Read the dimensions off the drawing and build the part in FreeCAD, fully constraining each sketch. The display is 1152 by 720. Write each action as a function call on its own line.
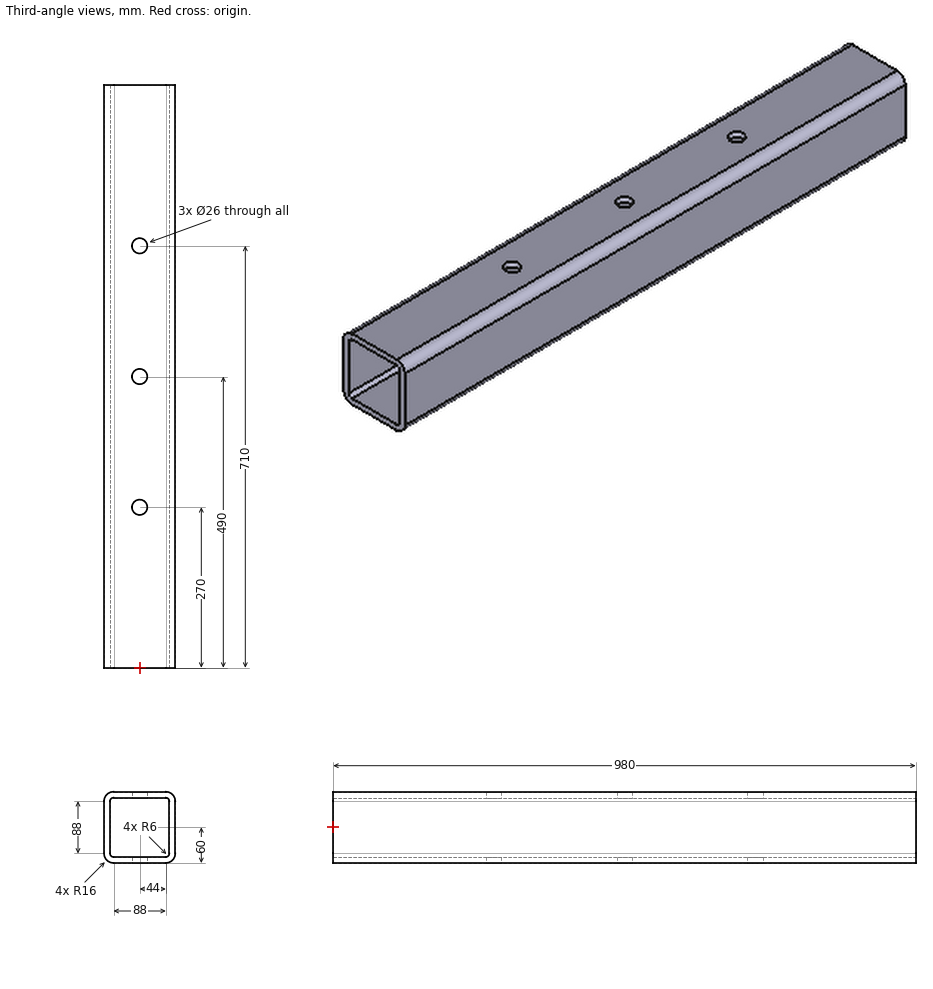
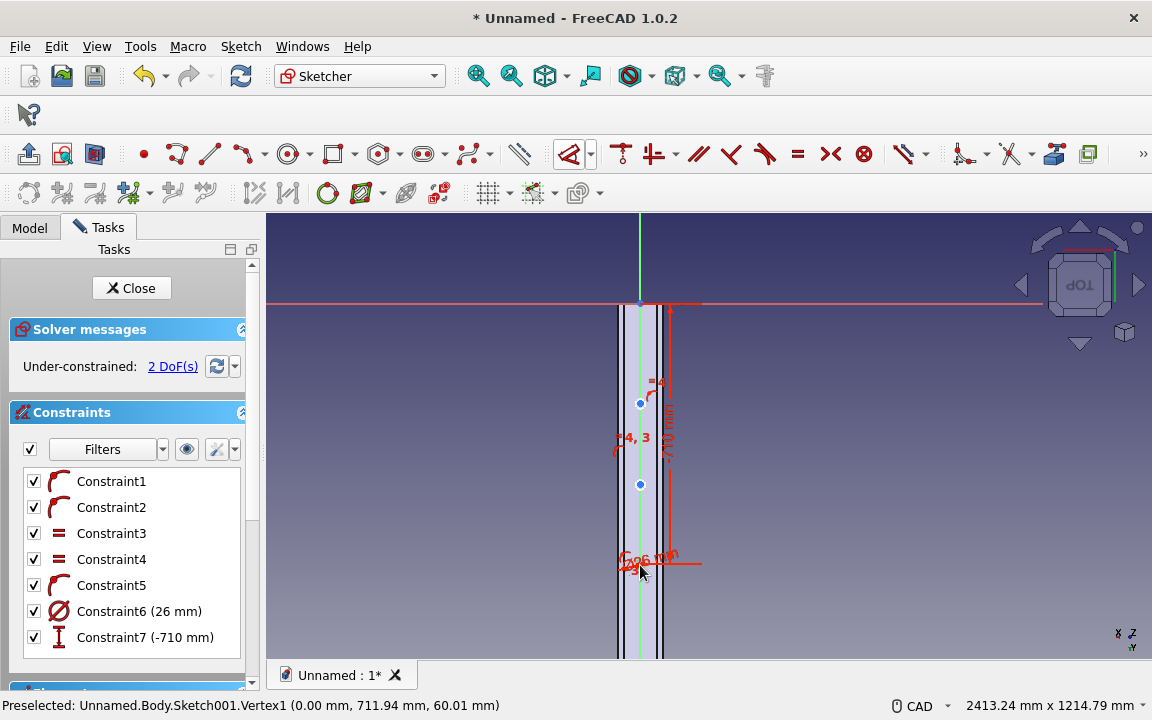
click(640, 485)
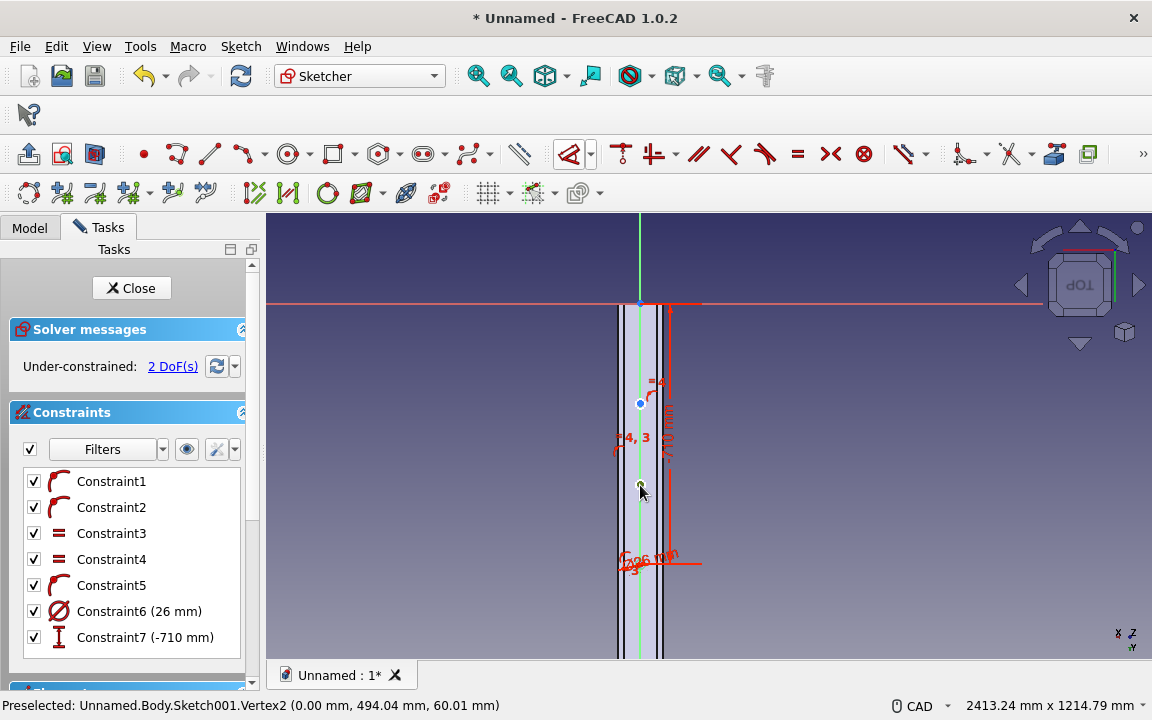
key(i)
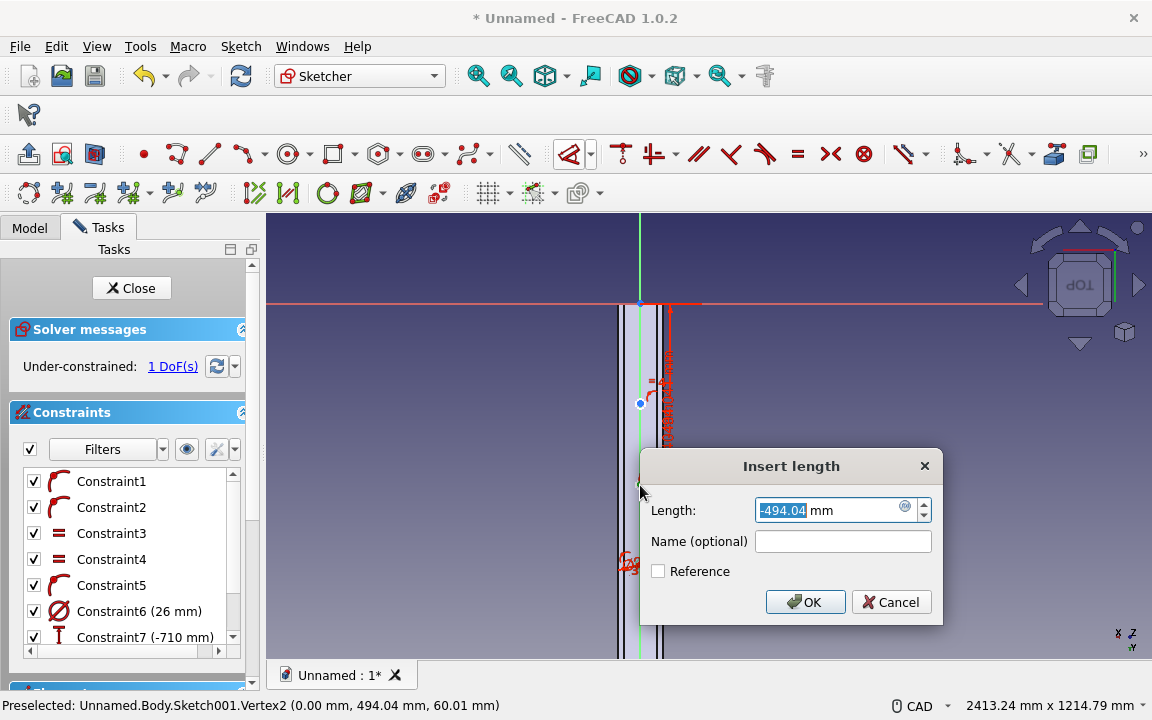
text(-490)
key(Return)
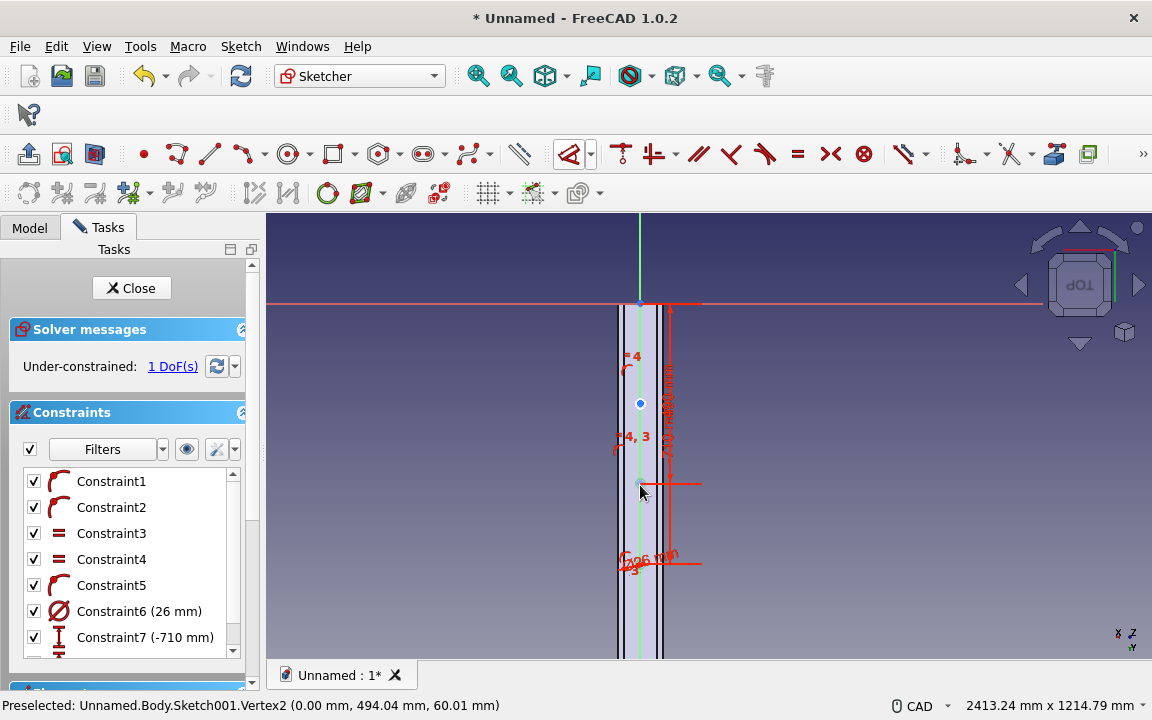
click(640, 404)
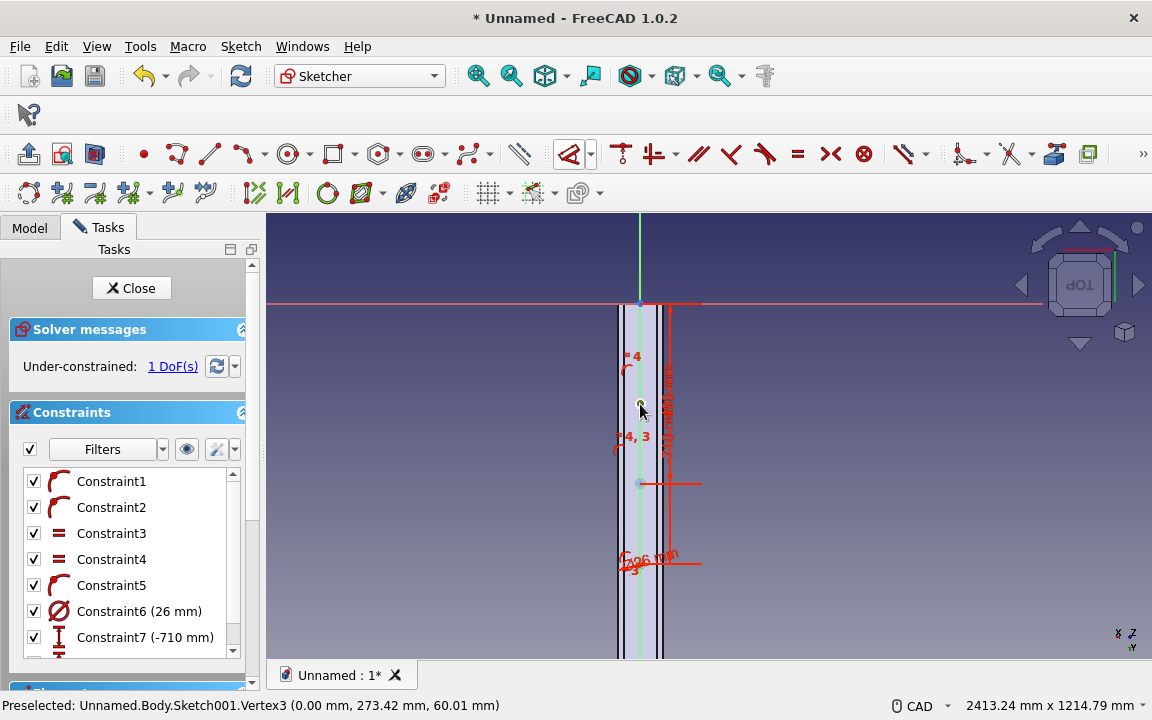
click(590, 154)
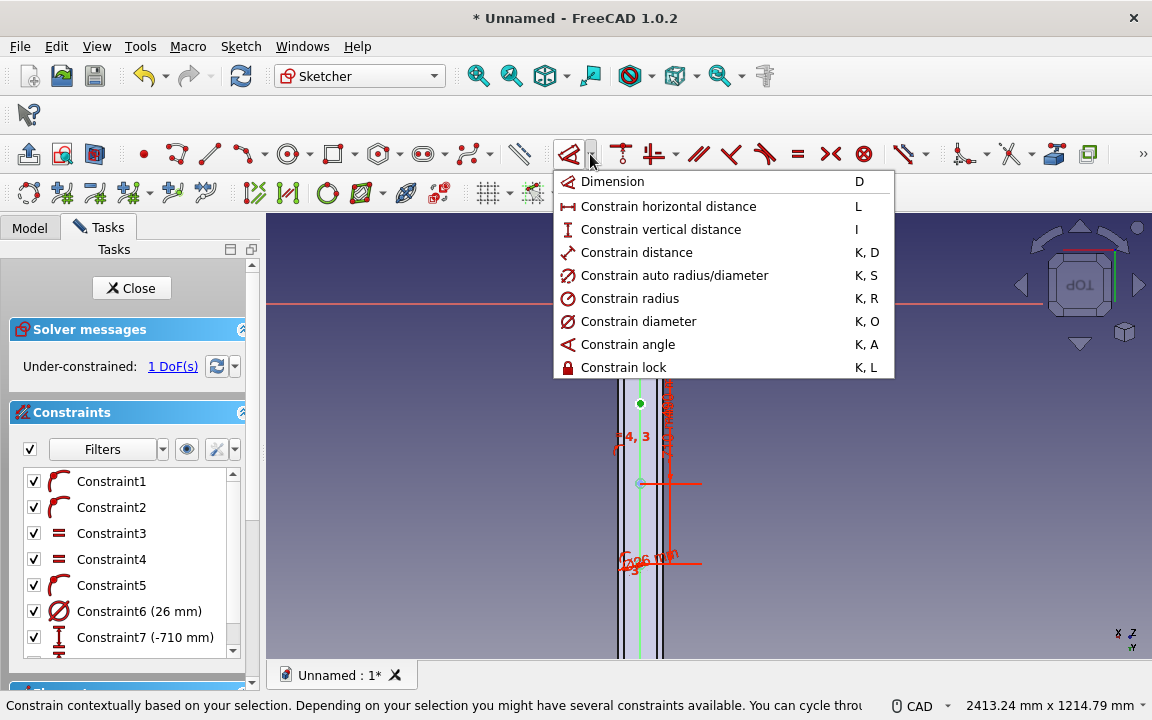
click(724, 230)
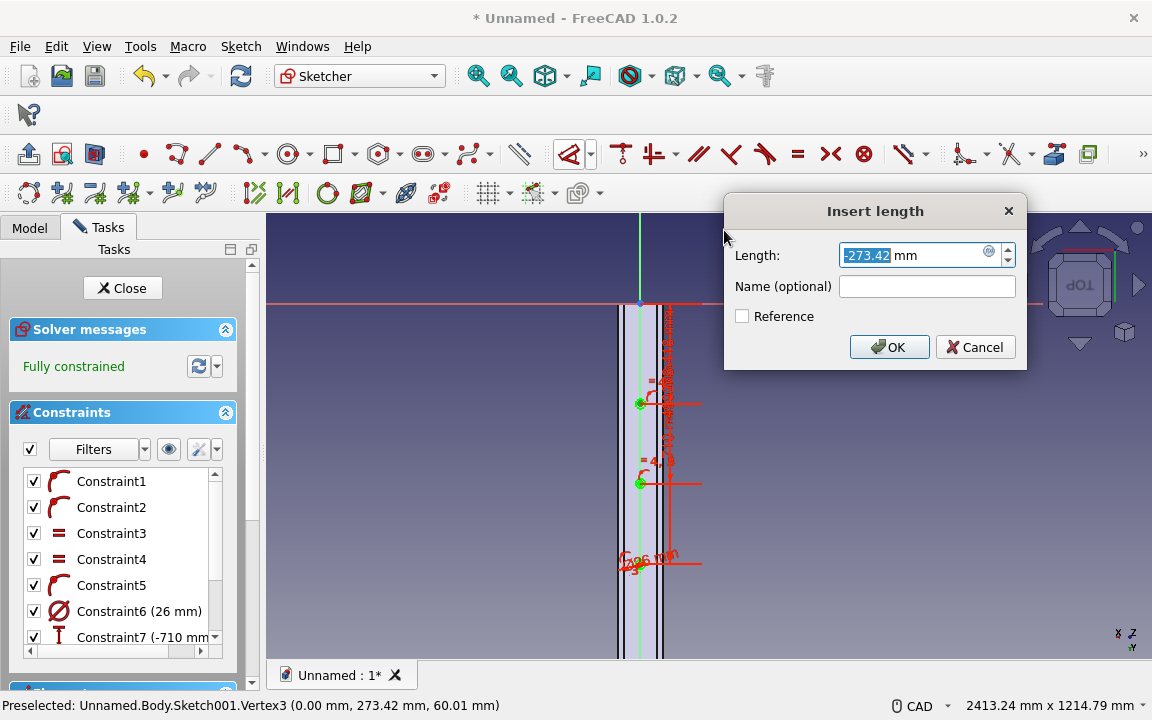
text(-270)
key(Return)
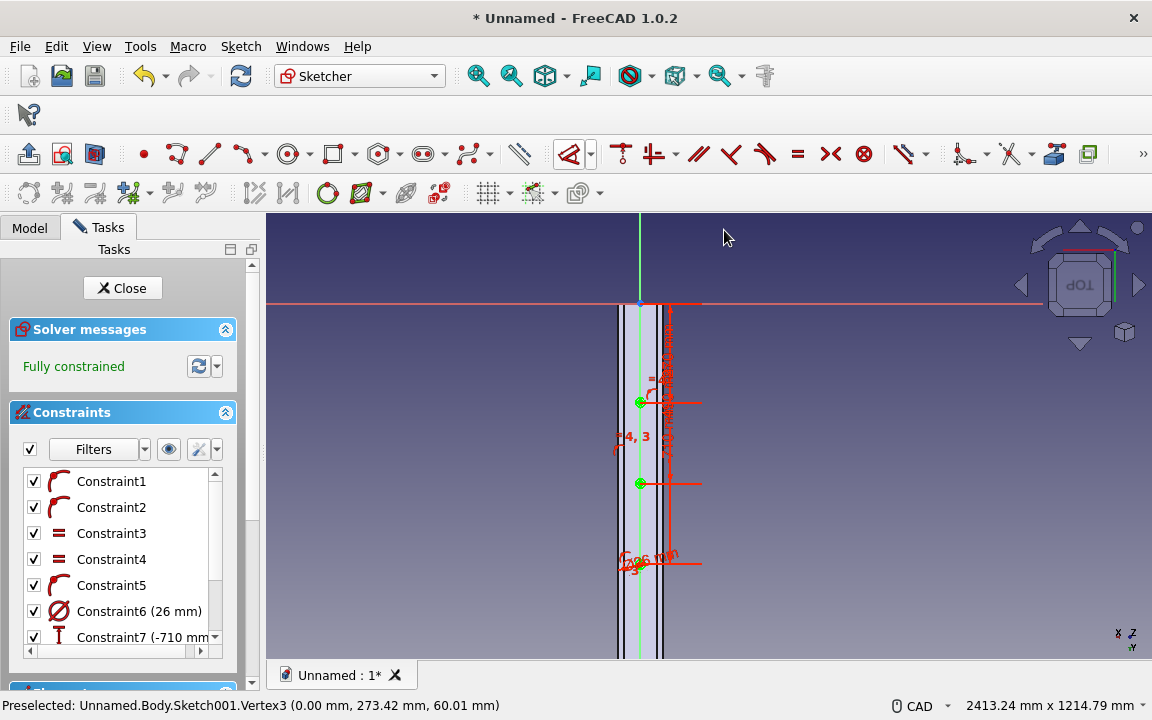
click(123, 288)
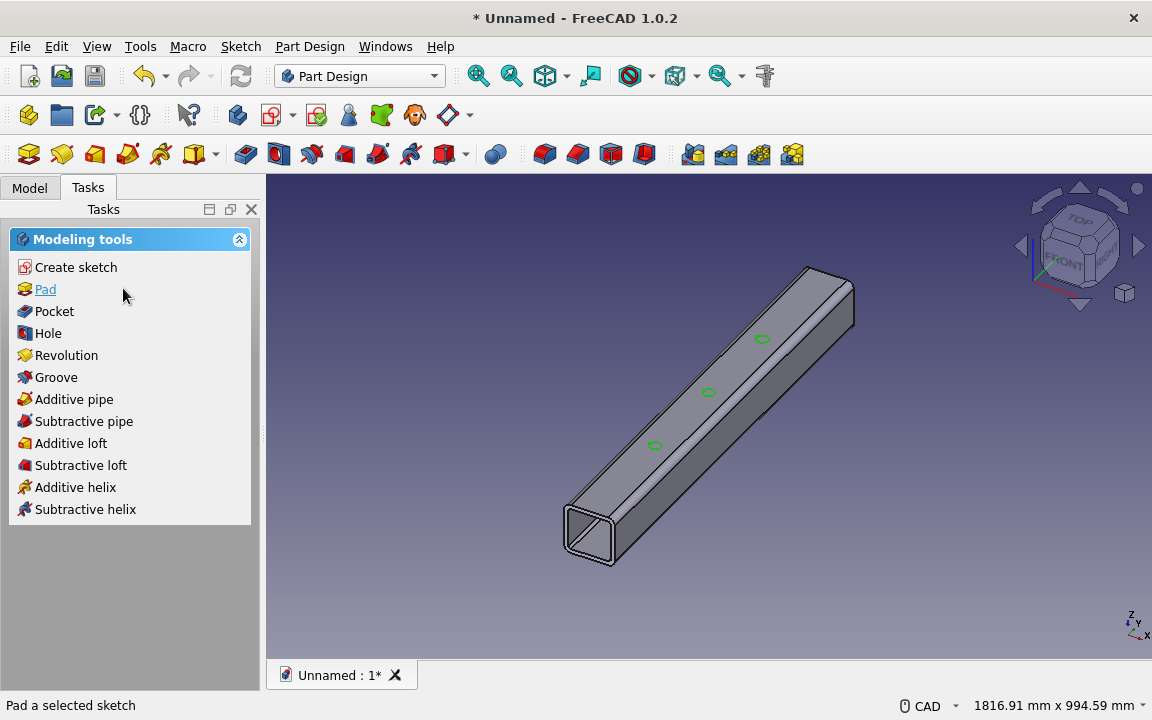
click(279, 154)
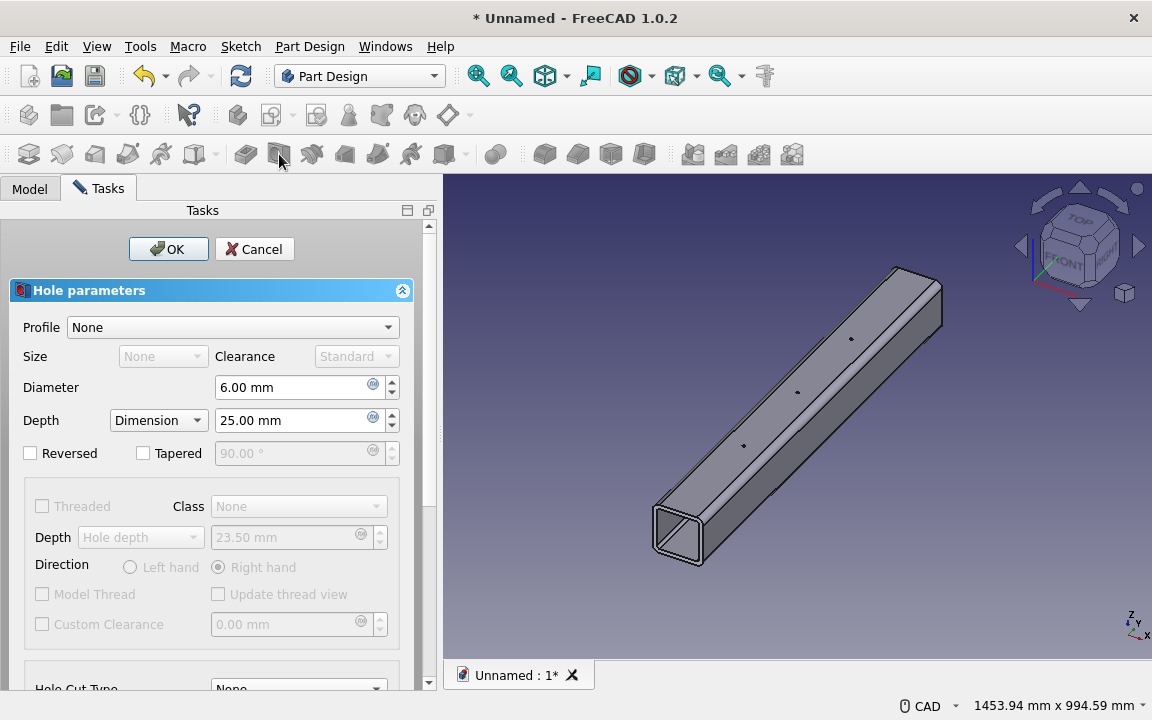
triple_click(300, 388)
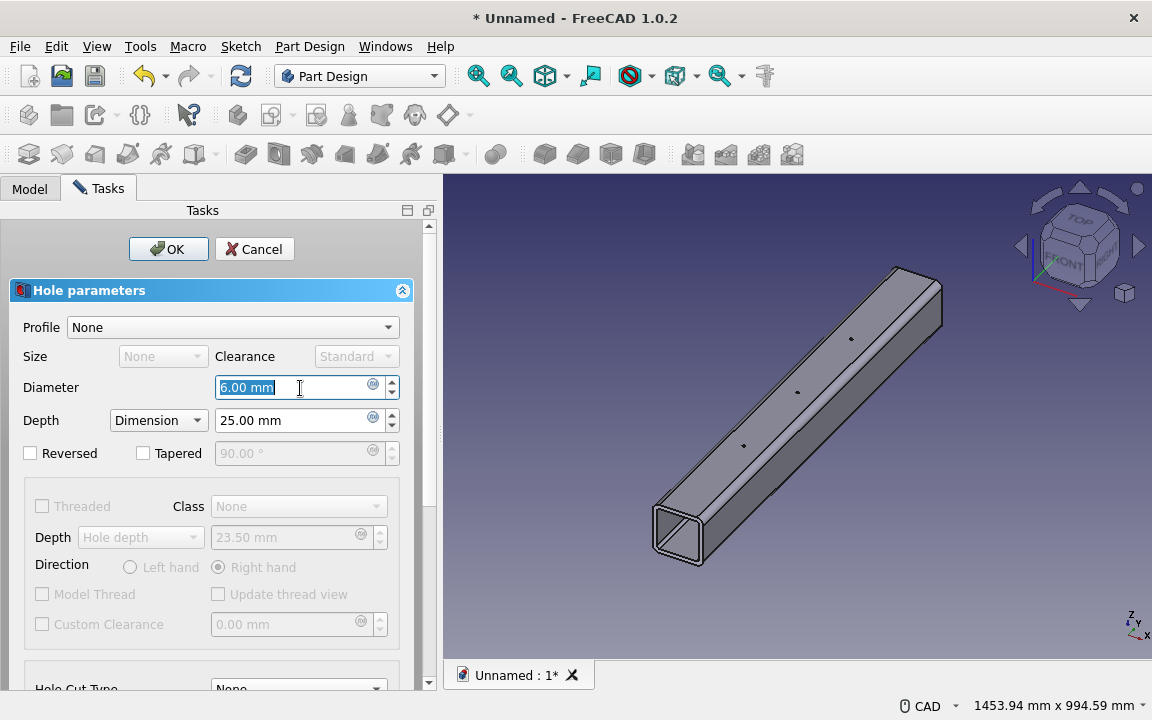
text(26)
key(Tab)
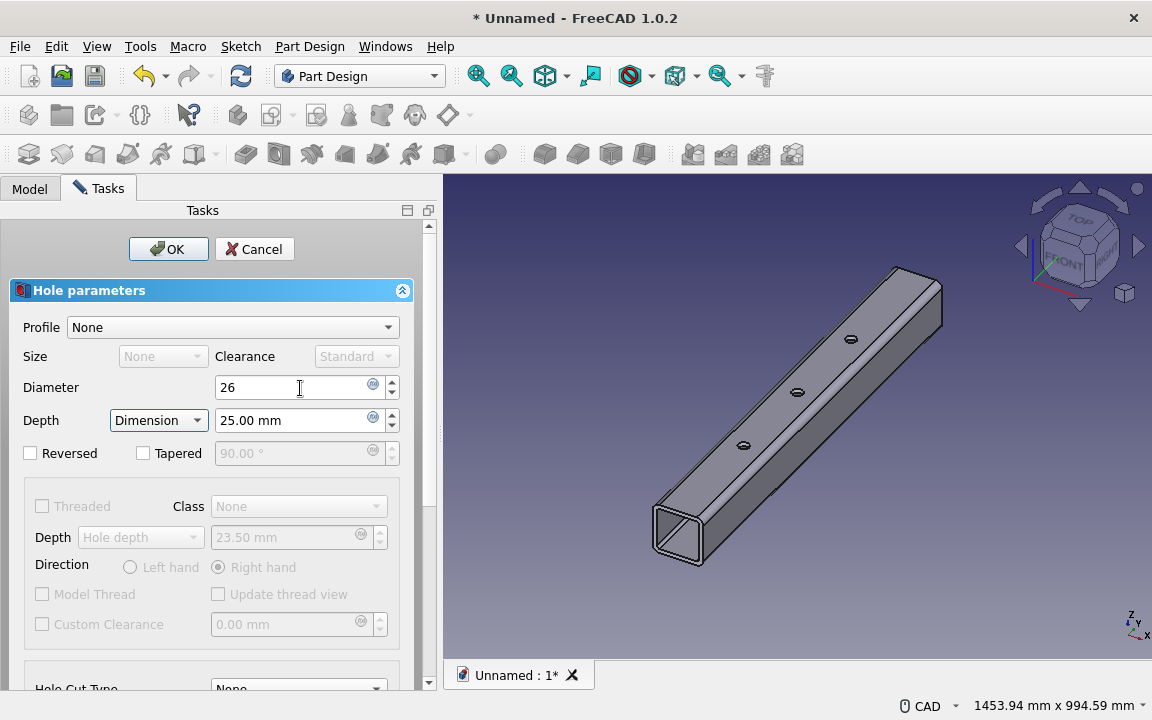
click(160, 420)